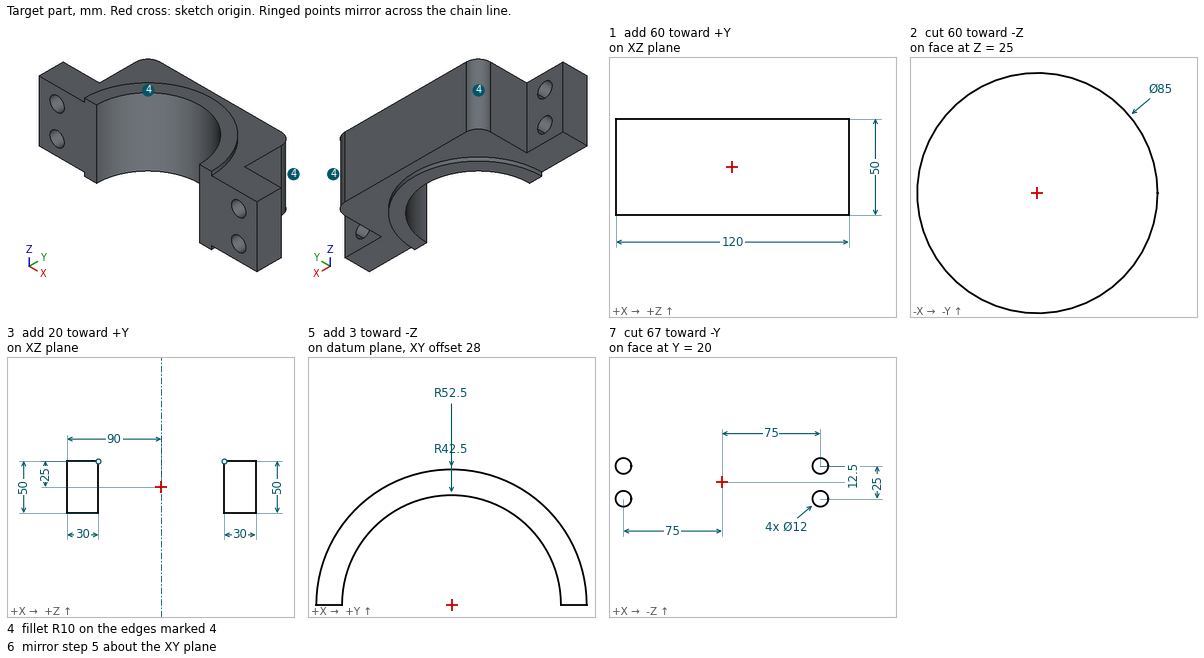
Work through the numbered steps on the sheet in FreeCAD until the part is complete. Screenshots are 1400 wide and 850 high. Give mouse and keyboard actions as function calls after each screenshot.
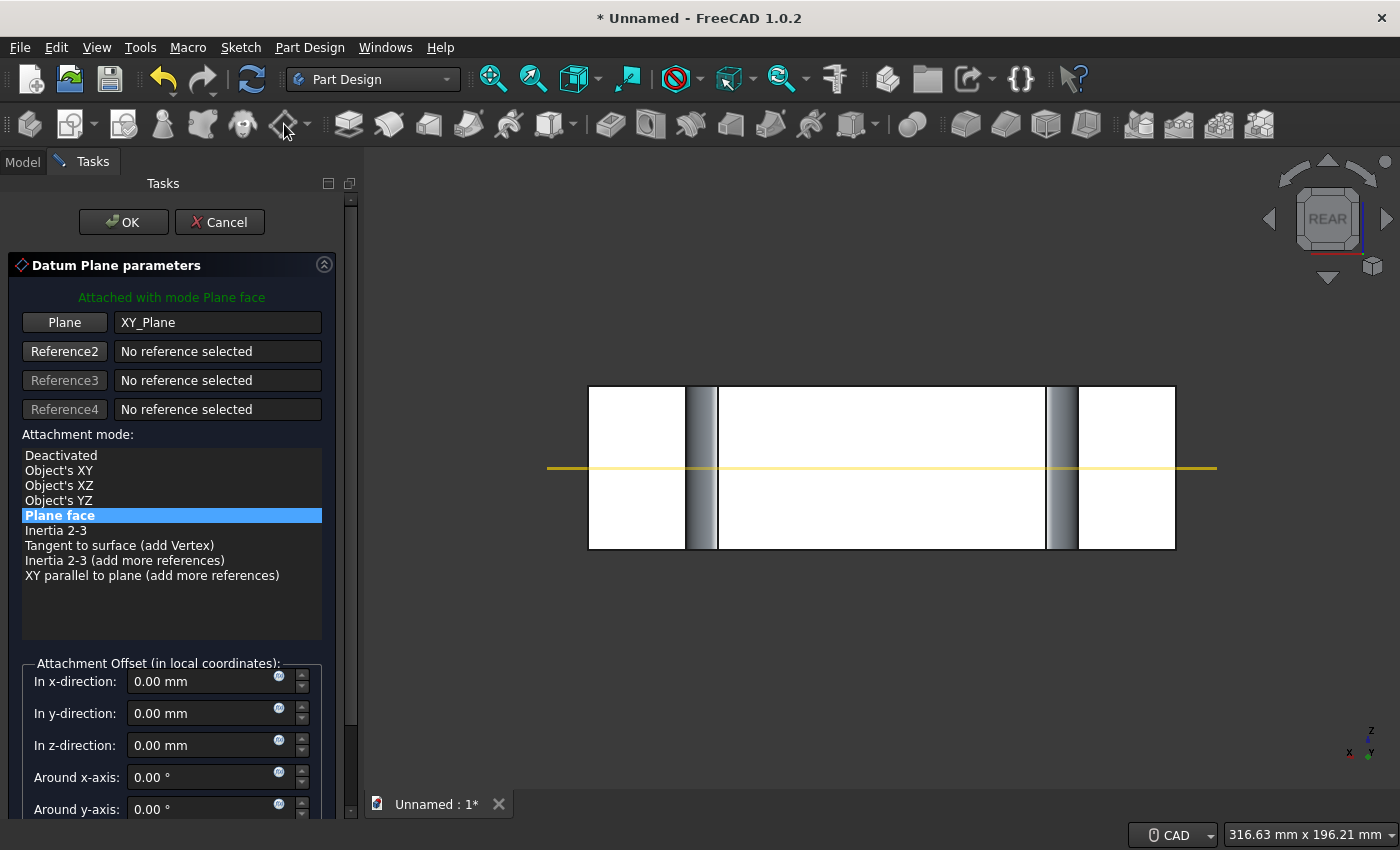
triple_click(210, 745)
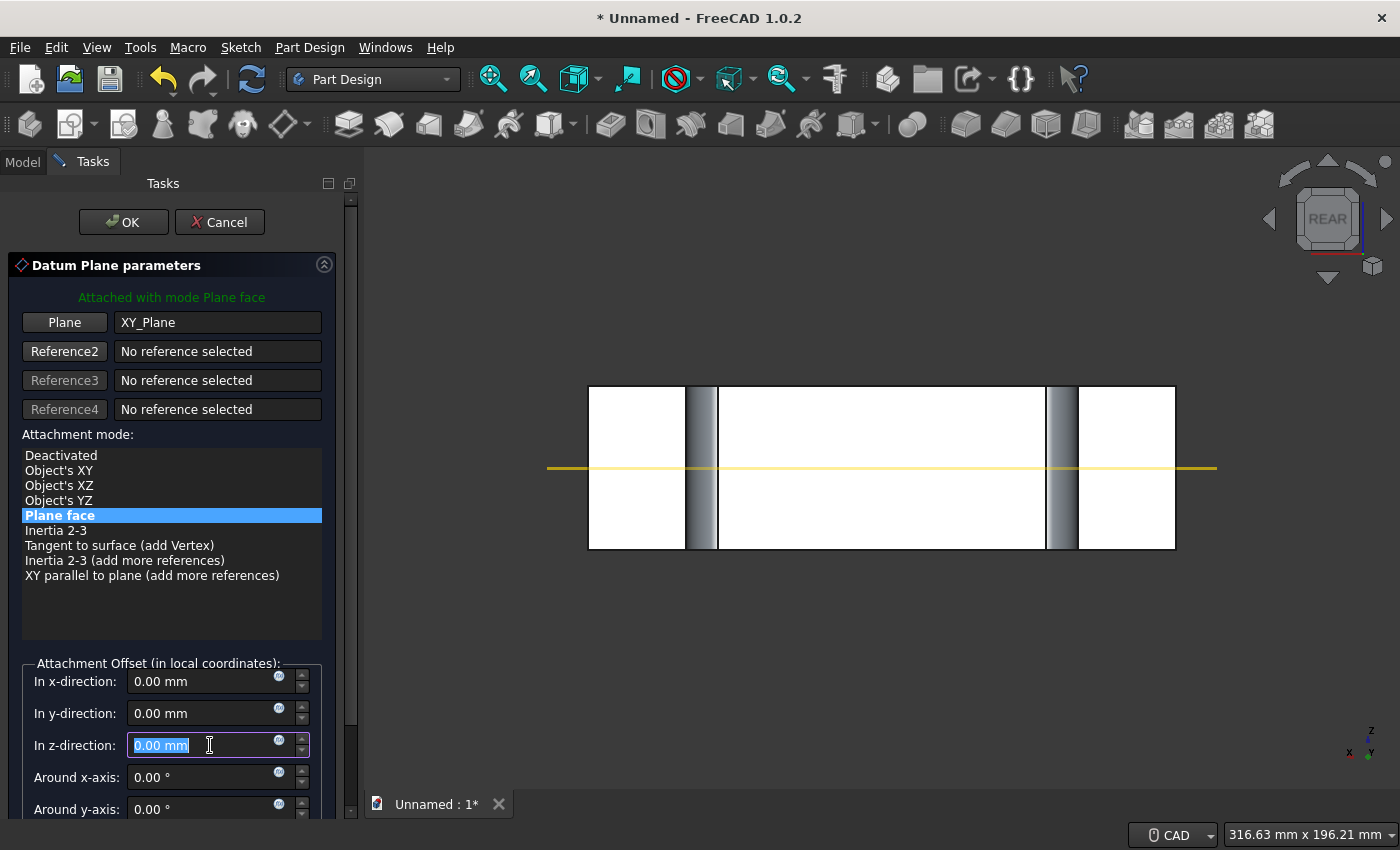
text(28)
key(Tab)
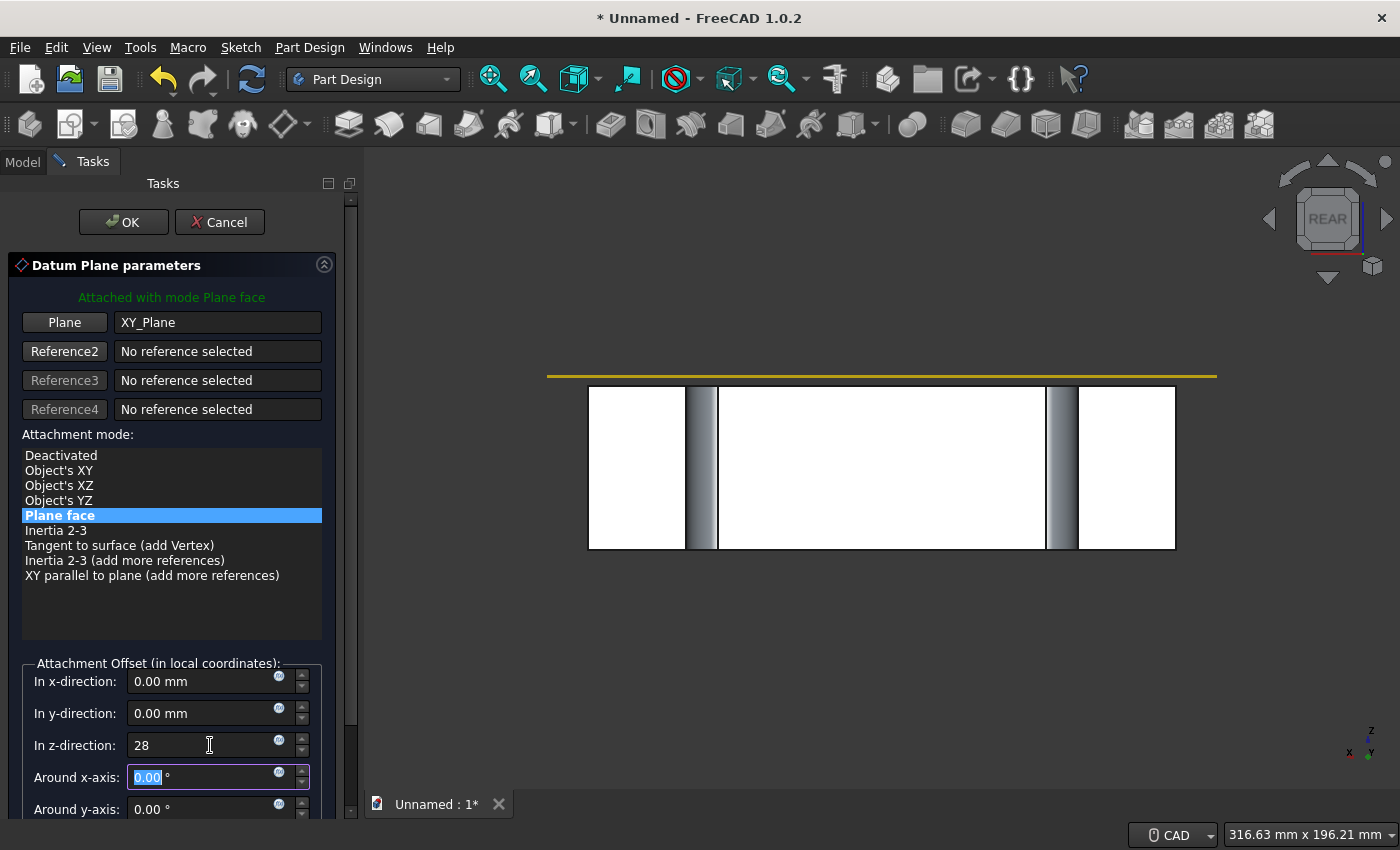
click(124, 222)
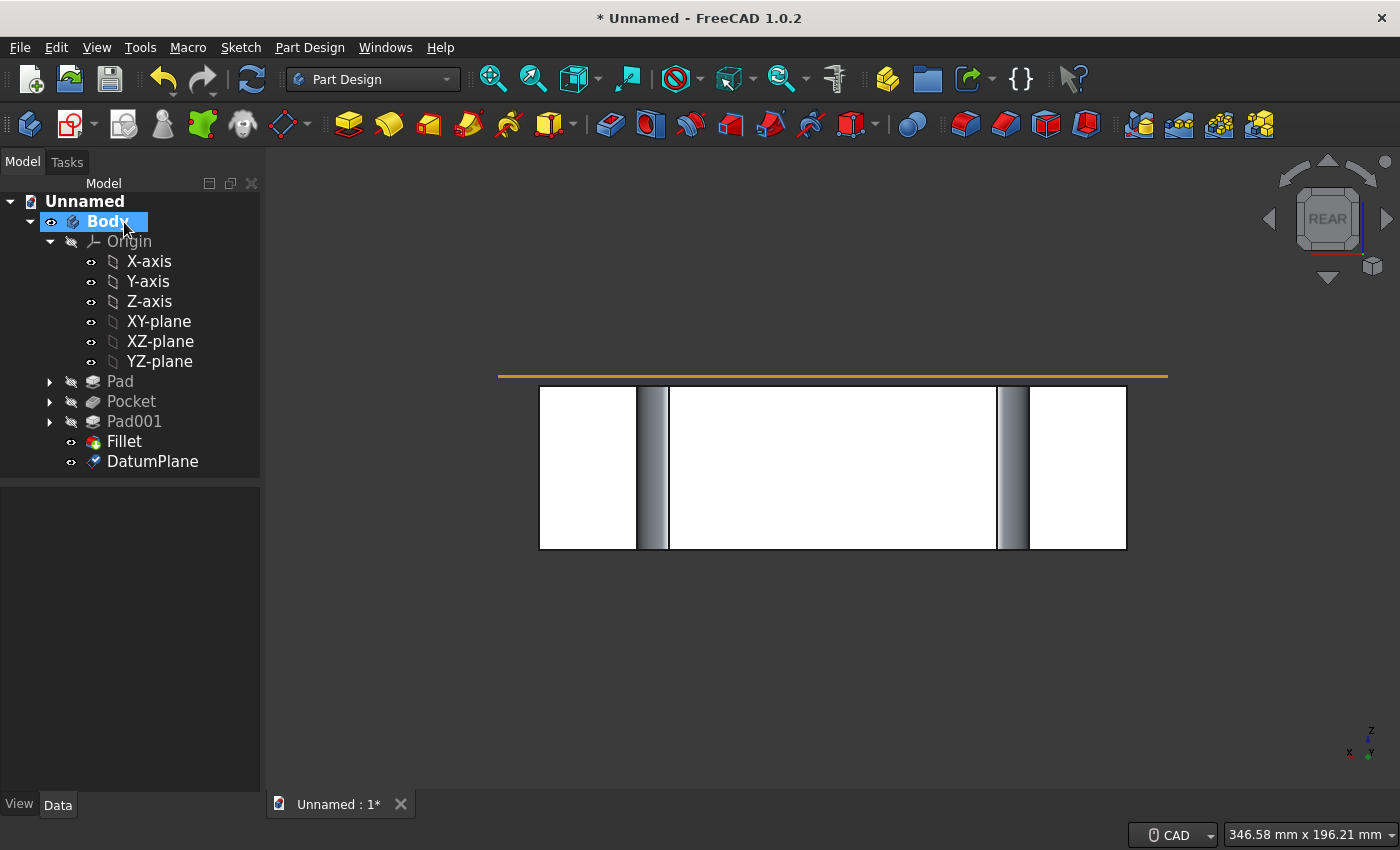
click(116, 462)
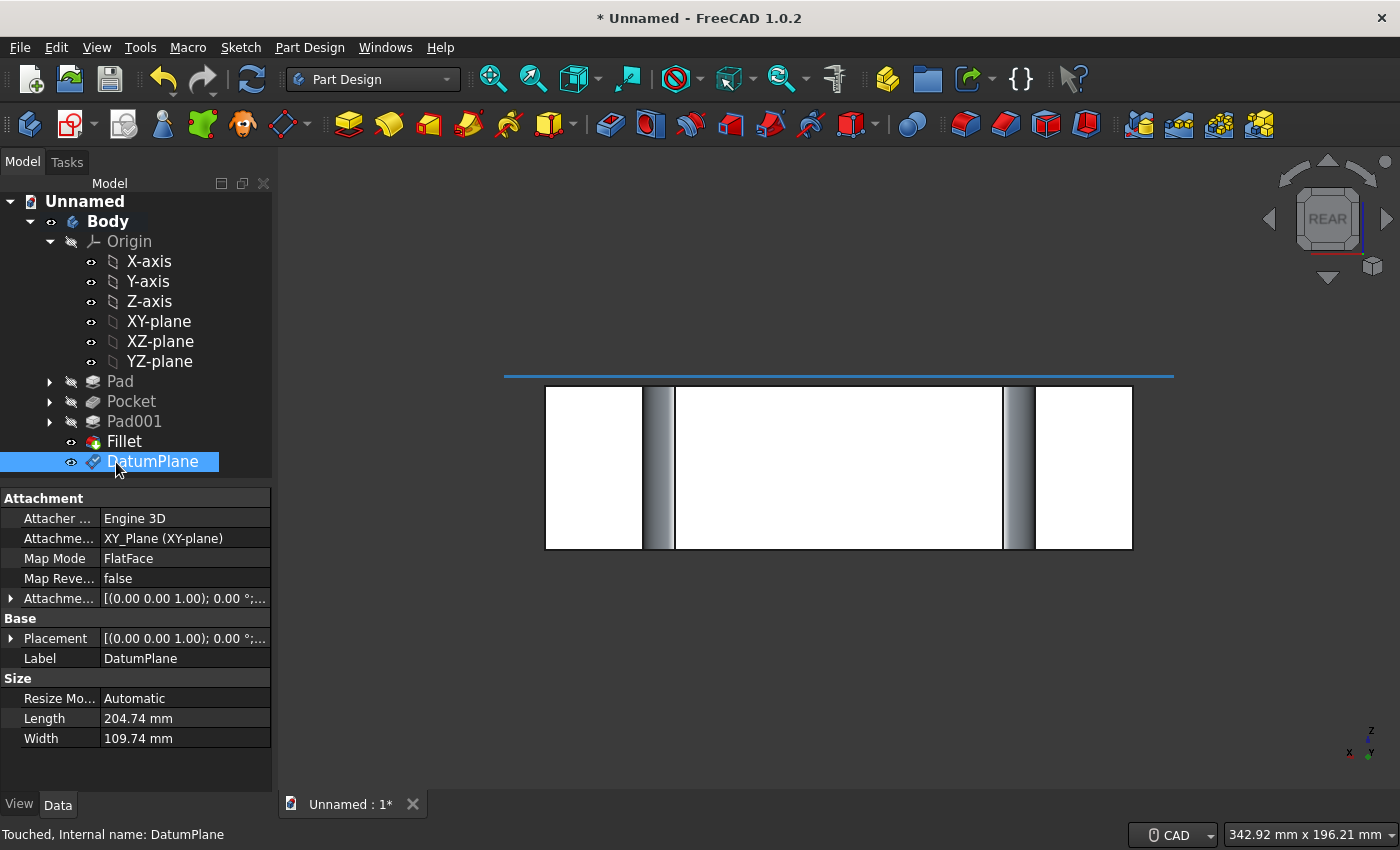
click(70, 124)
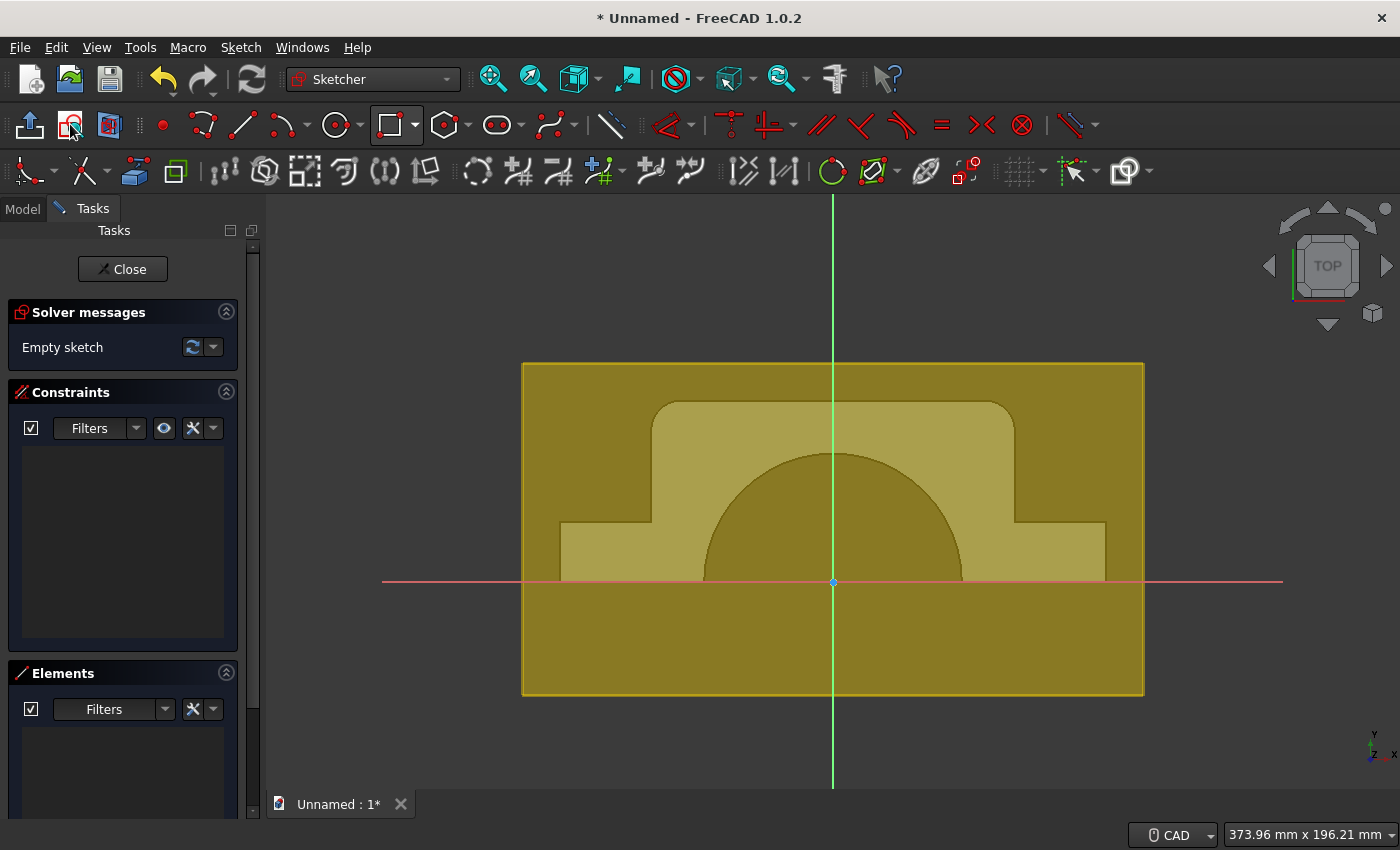
scroll(889, 512, up, 4)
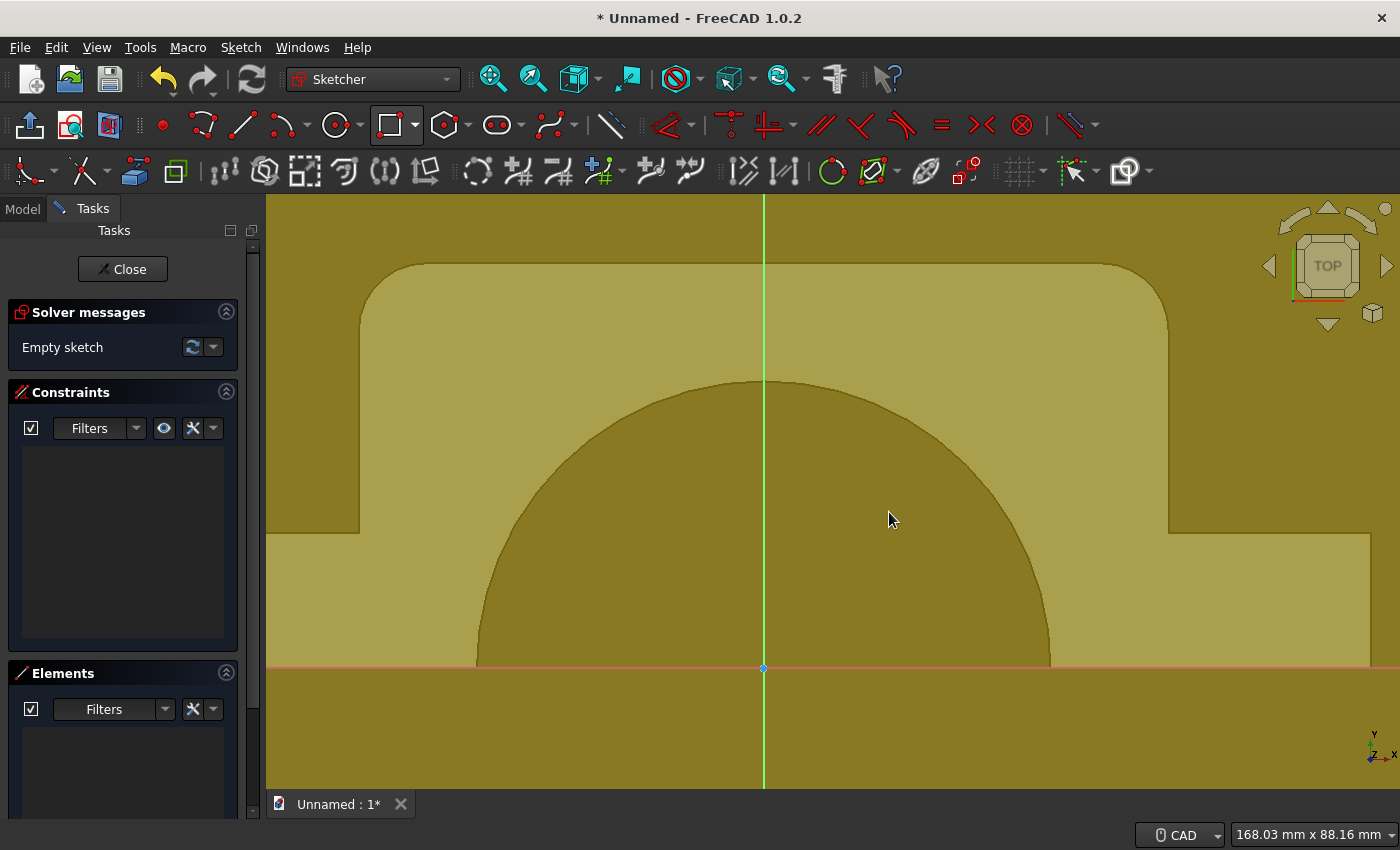
click(244, 126)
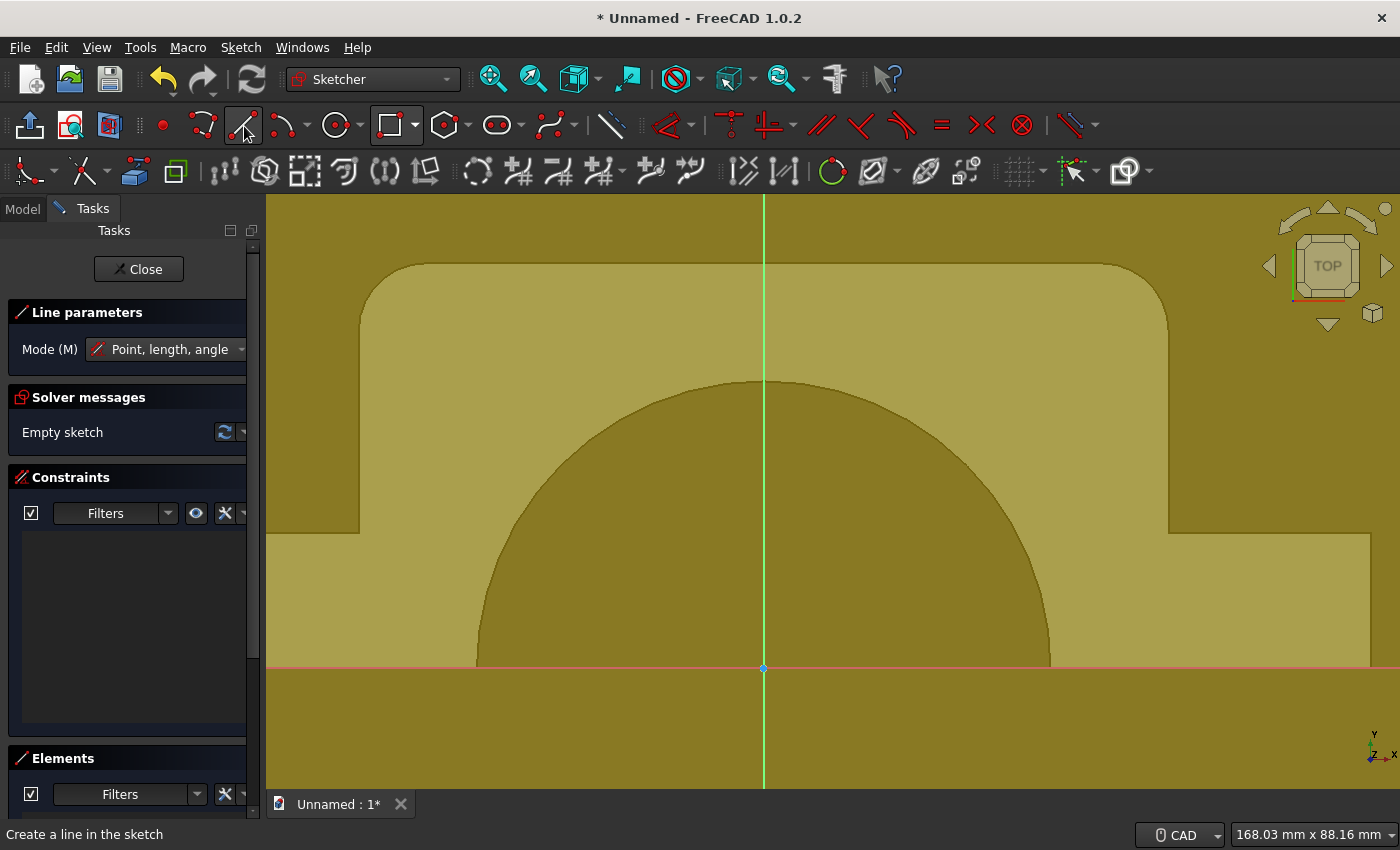
click(409, 668)
click(477, 659)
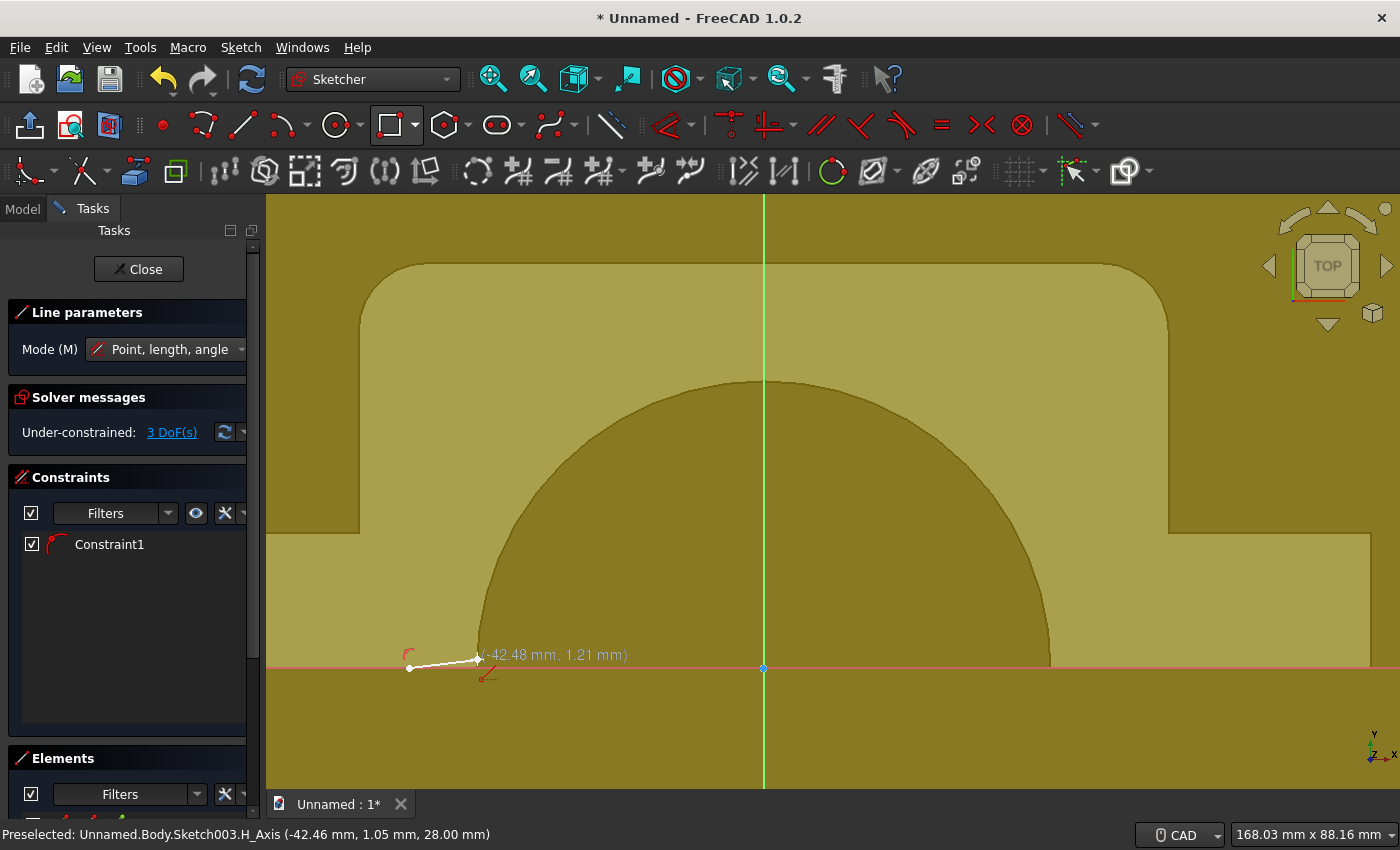
click(1051, 668)
click(1118, 659)